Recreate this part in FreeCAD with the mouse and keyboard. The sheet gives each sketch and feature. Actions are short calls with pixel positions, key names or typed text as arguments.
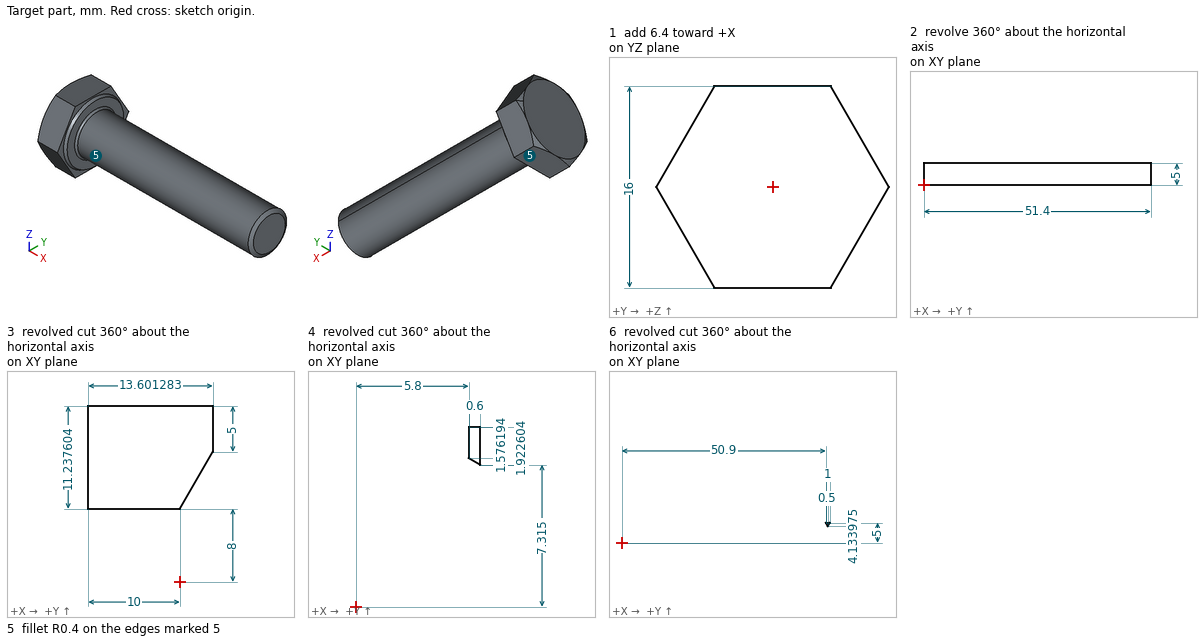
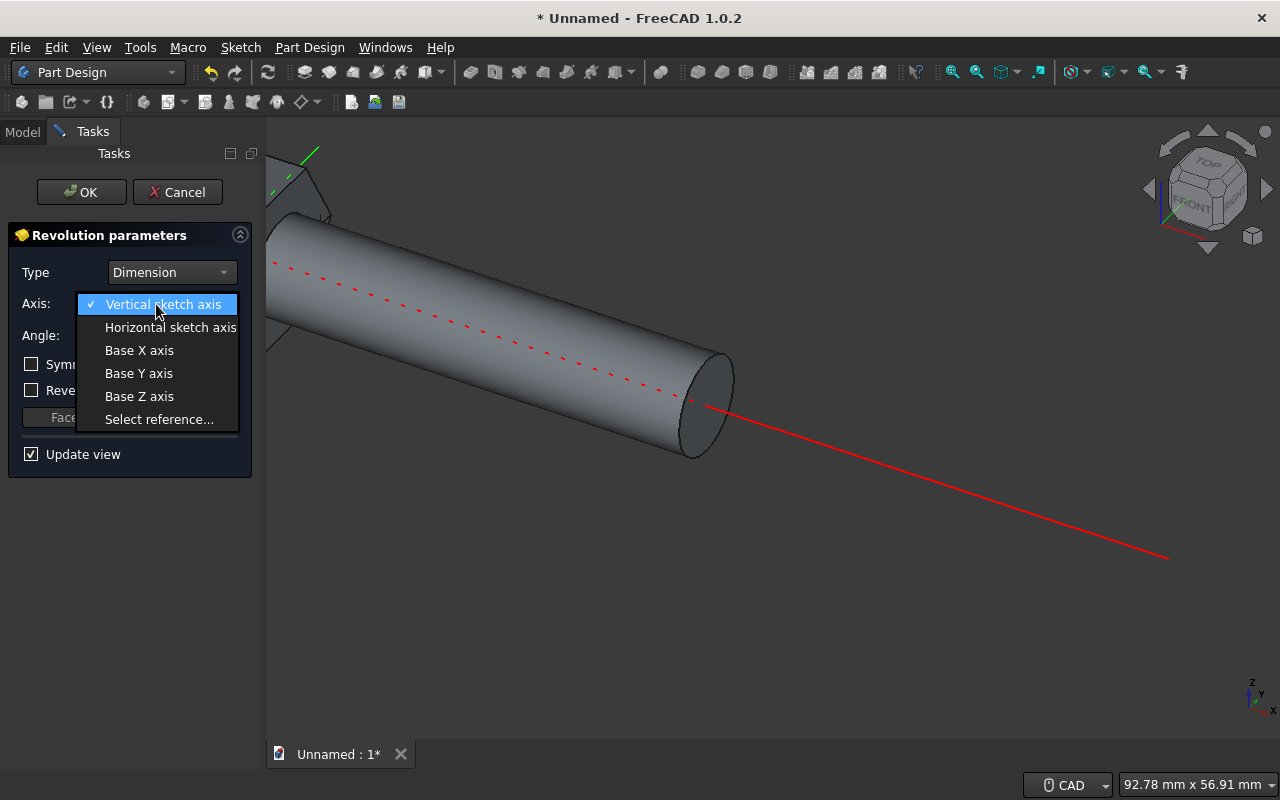
click(156, 328)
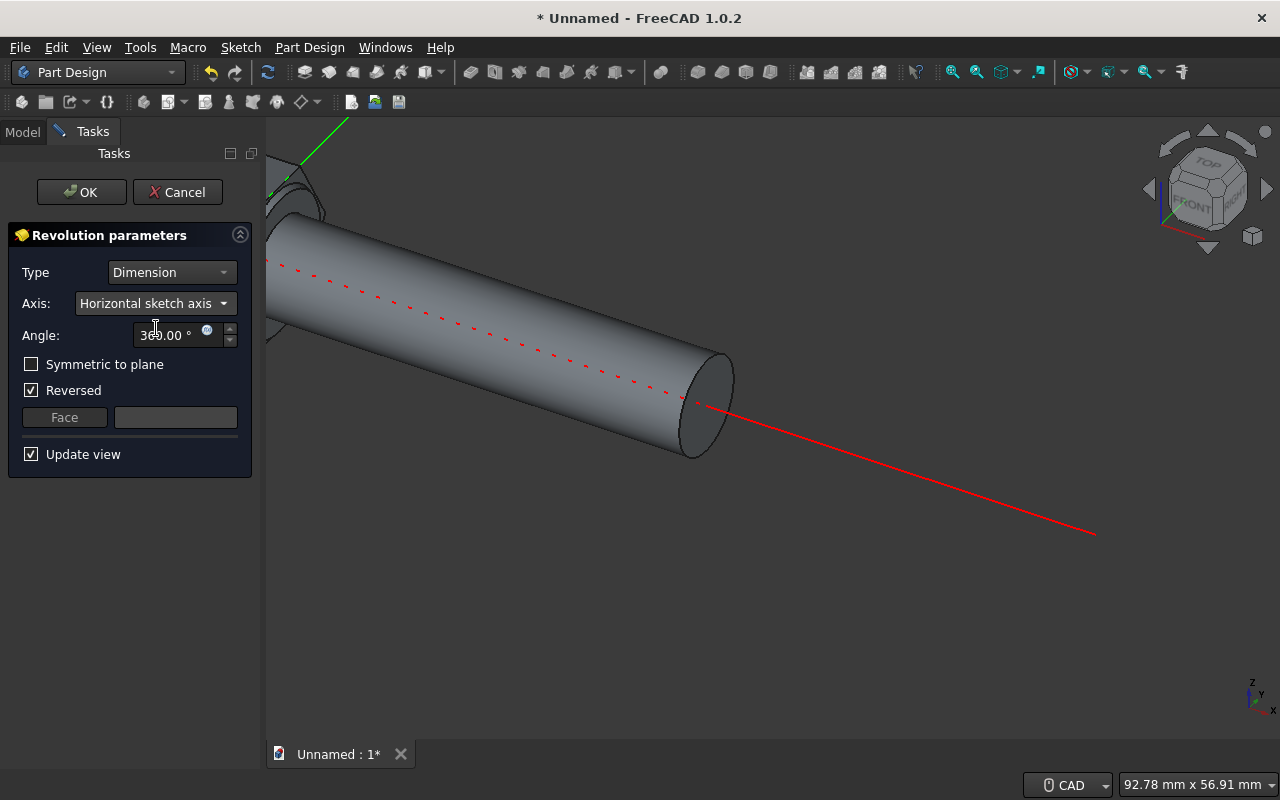
click(82, 192)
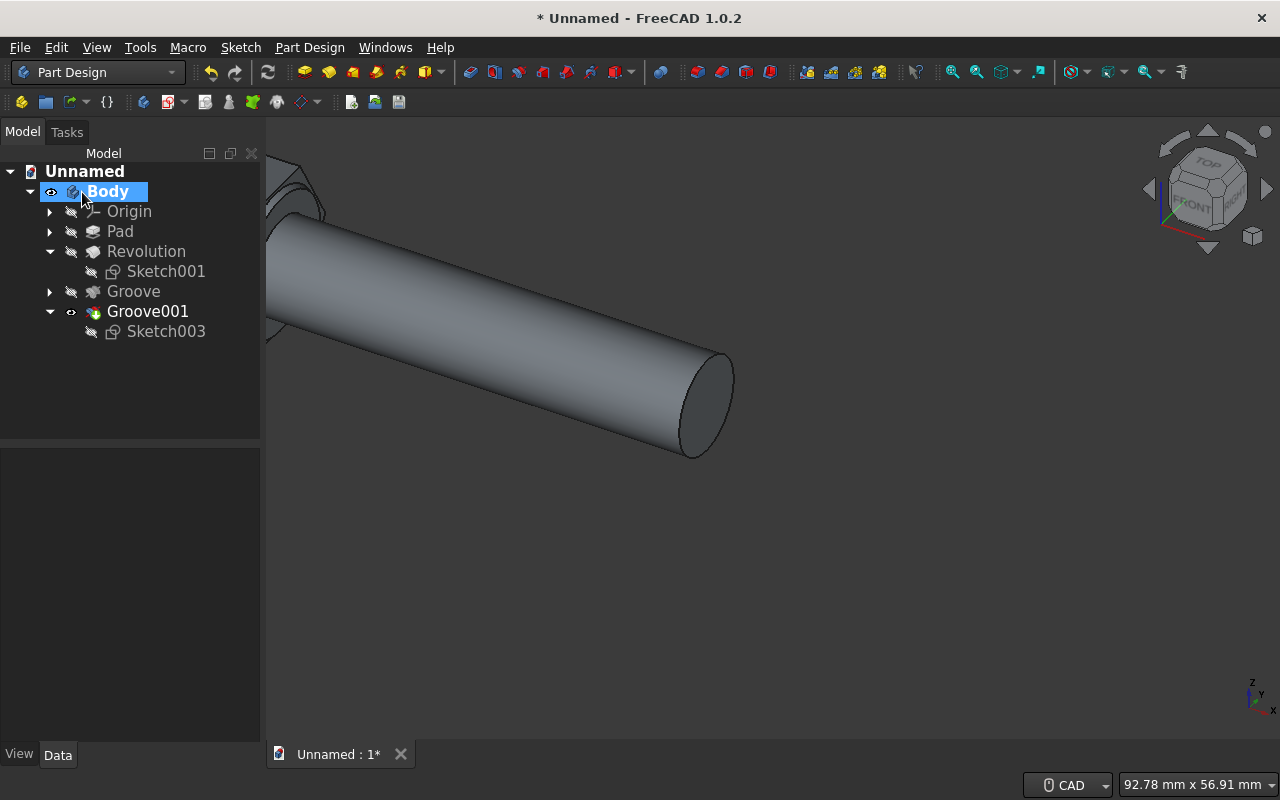
key(v)
key(f)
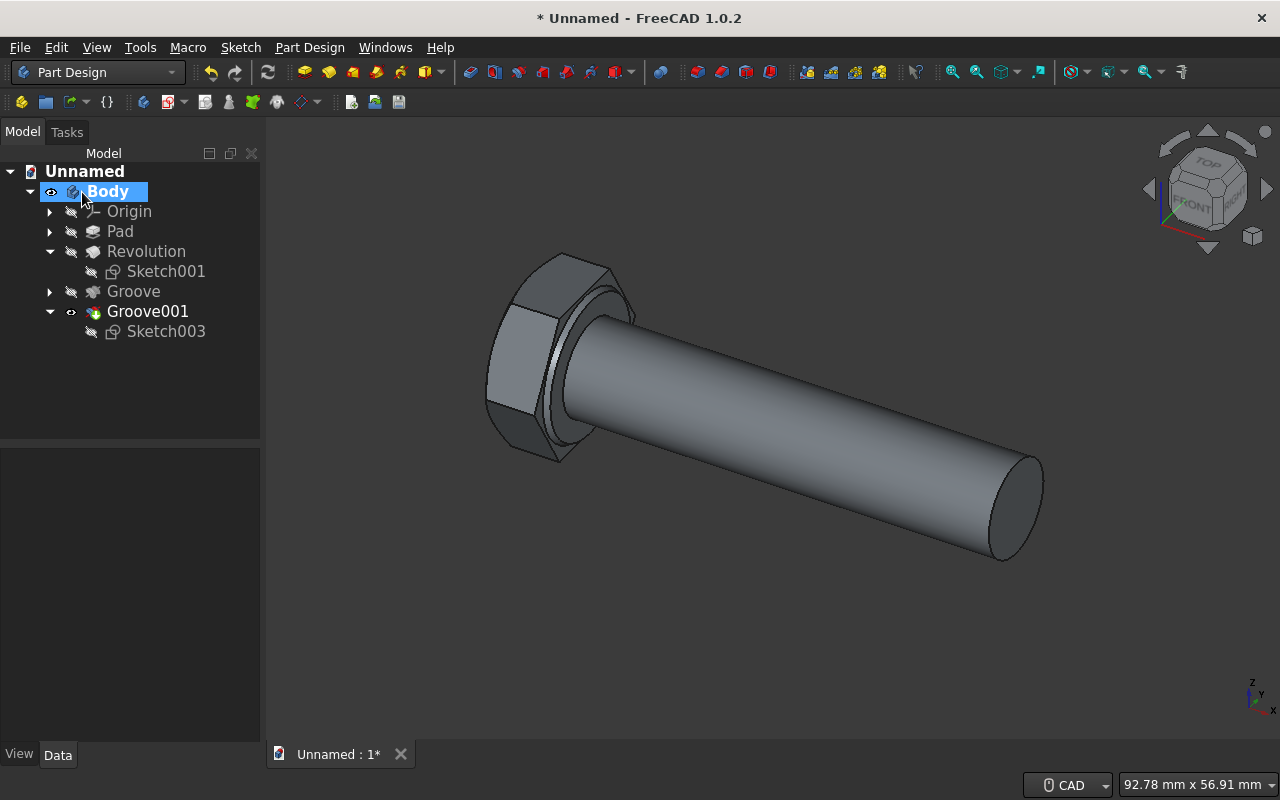
key(0)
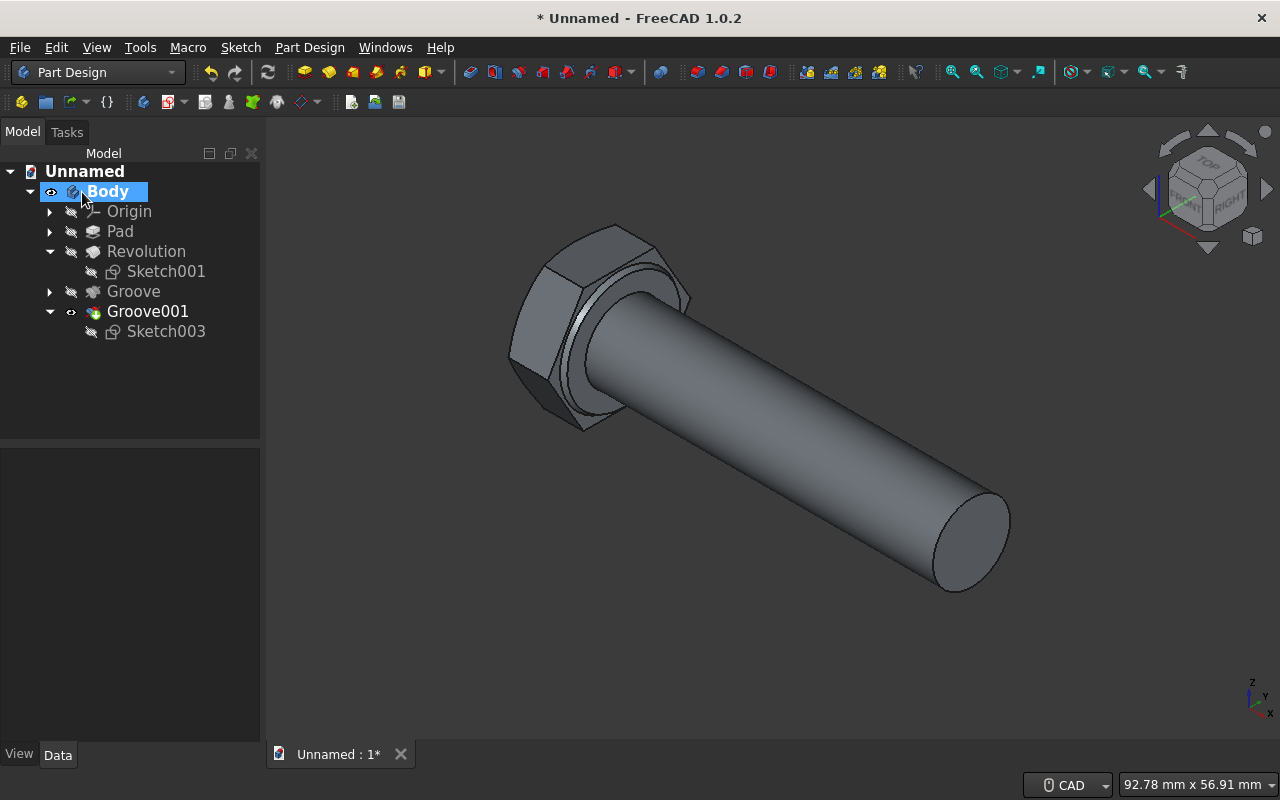
key(2)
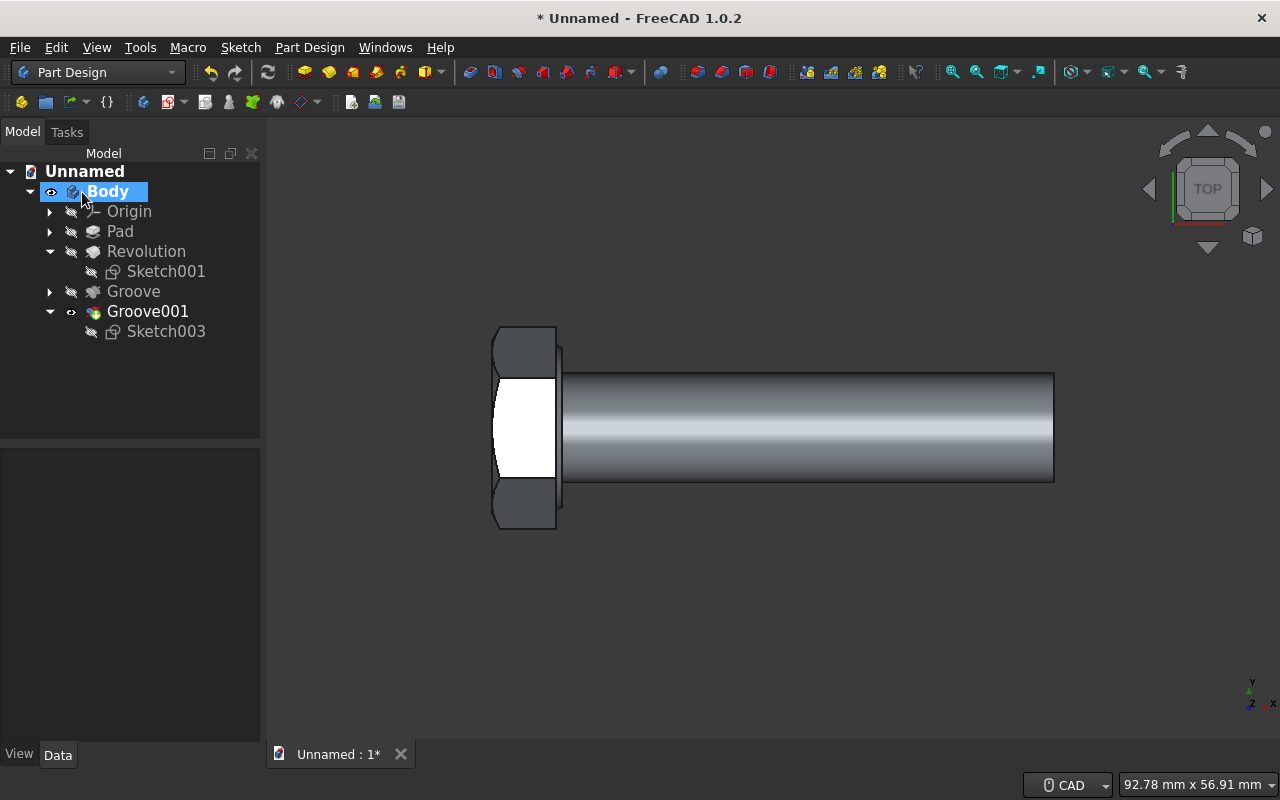
key(1)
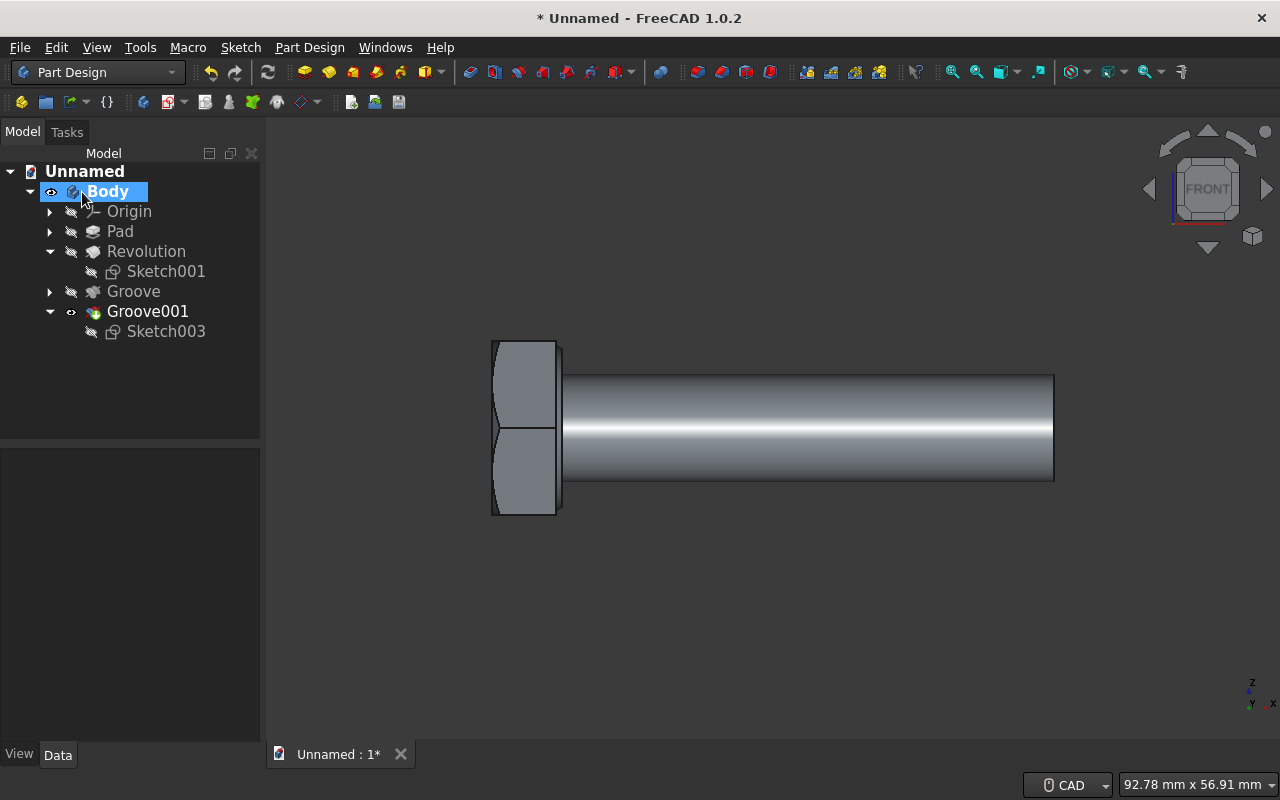
key(3)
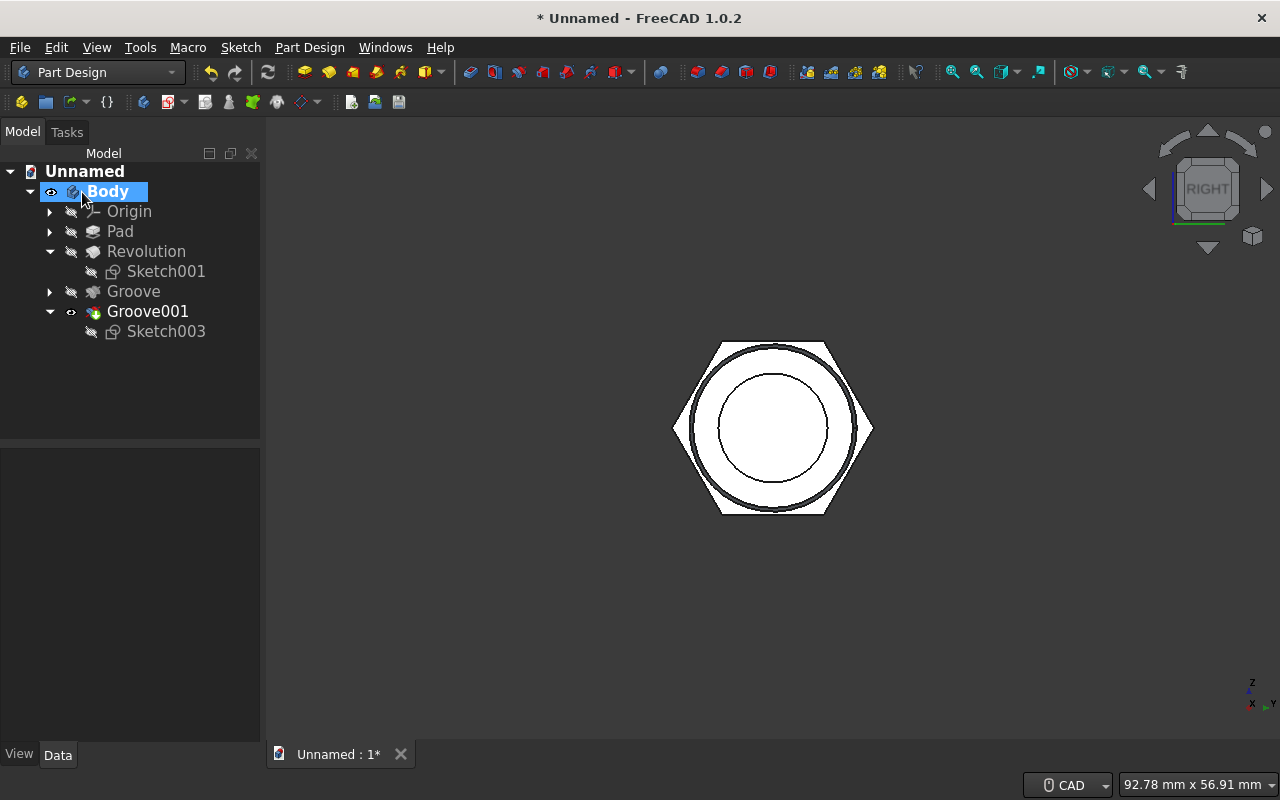
click(954, 72)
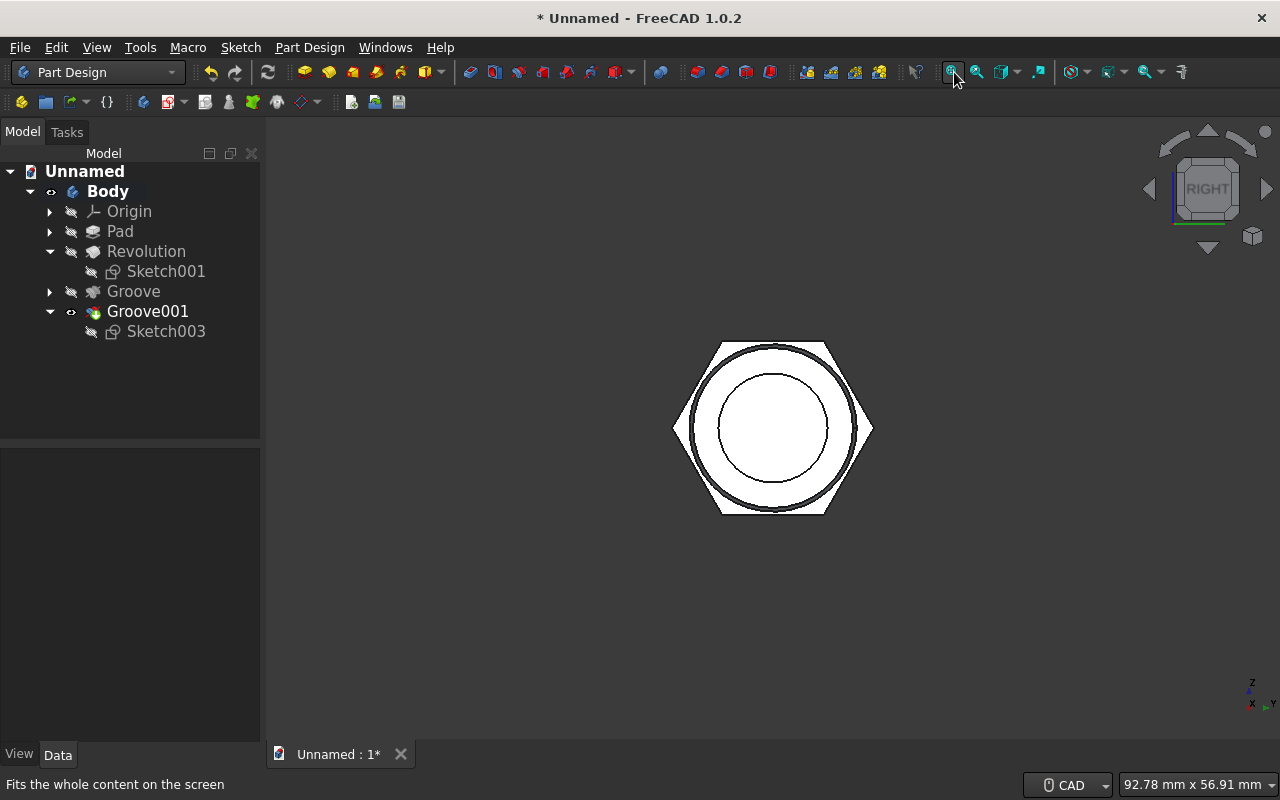
key(5)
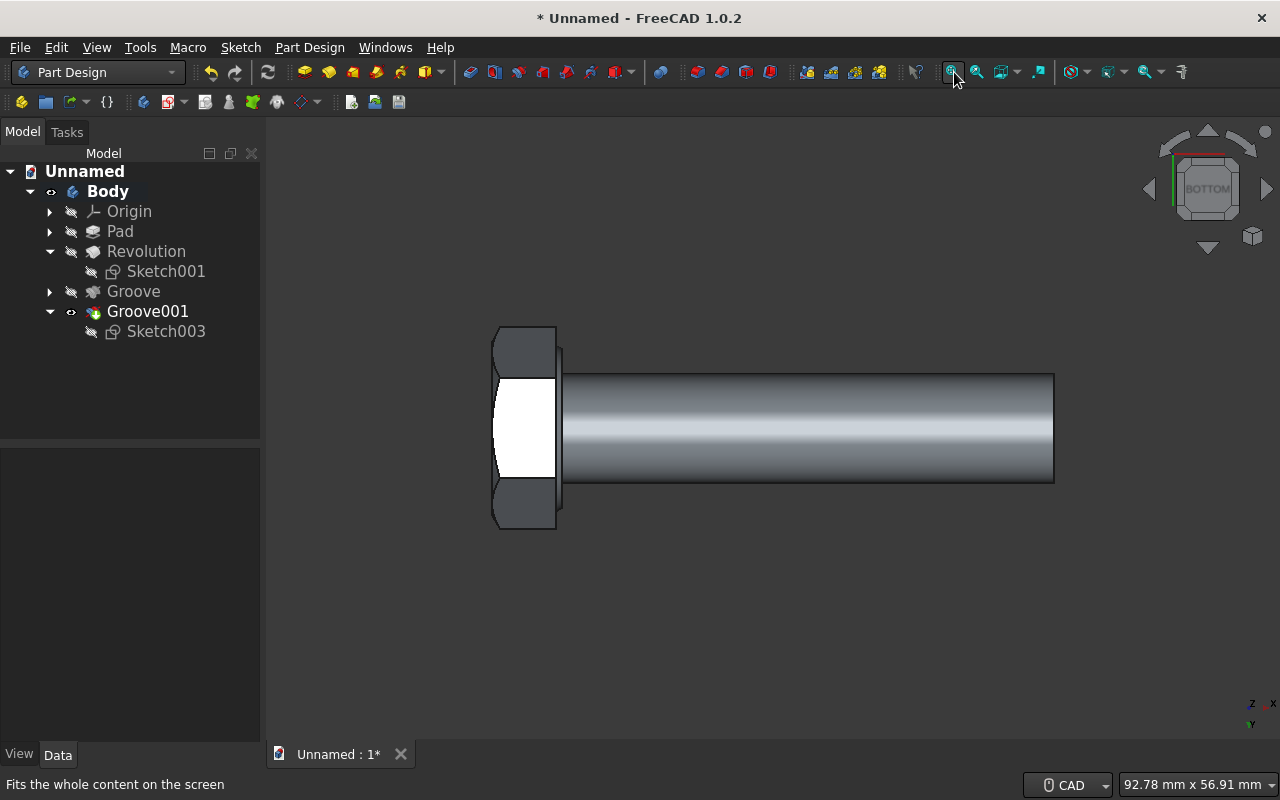
key(4)